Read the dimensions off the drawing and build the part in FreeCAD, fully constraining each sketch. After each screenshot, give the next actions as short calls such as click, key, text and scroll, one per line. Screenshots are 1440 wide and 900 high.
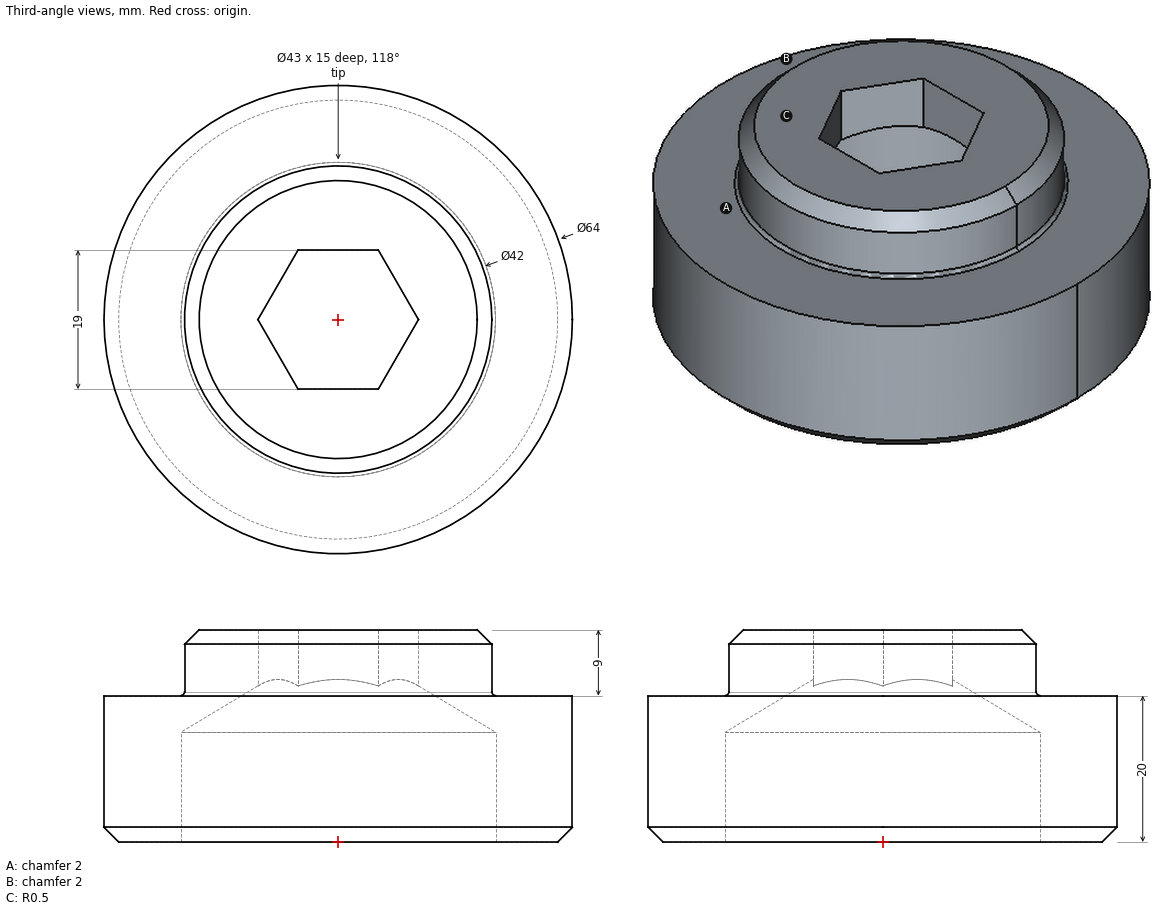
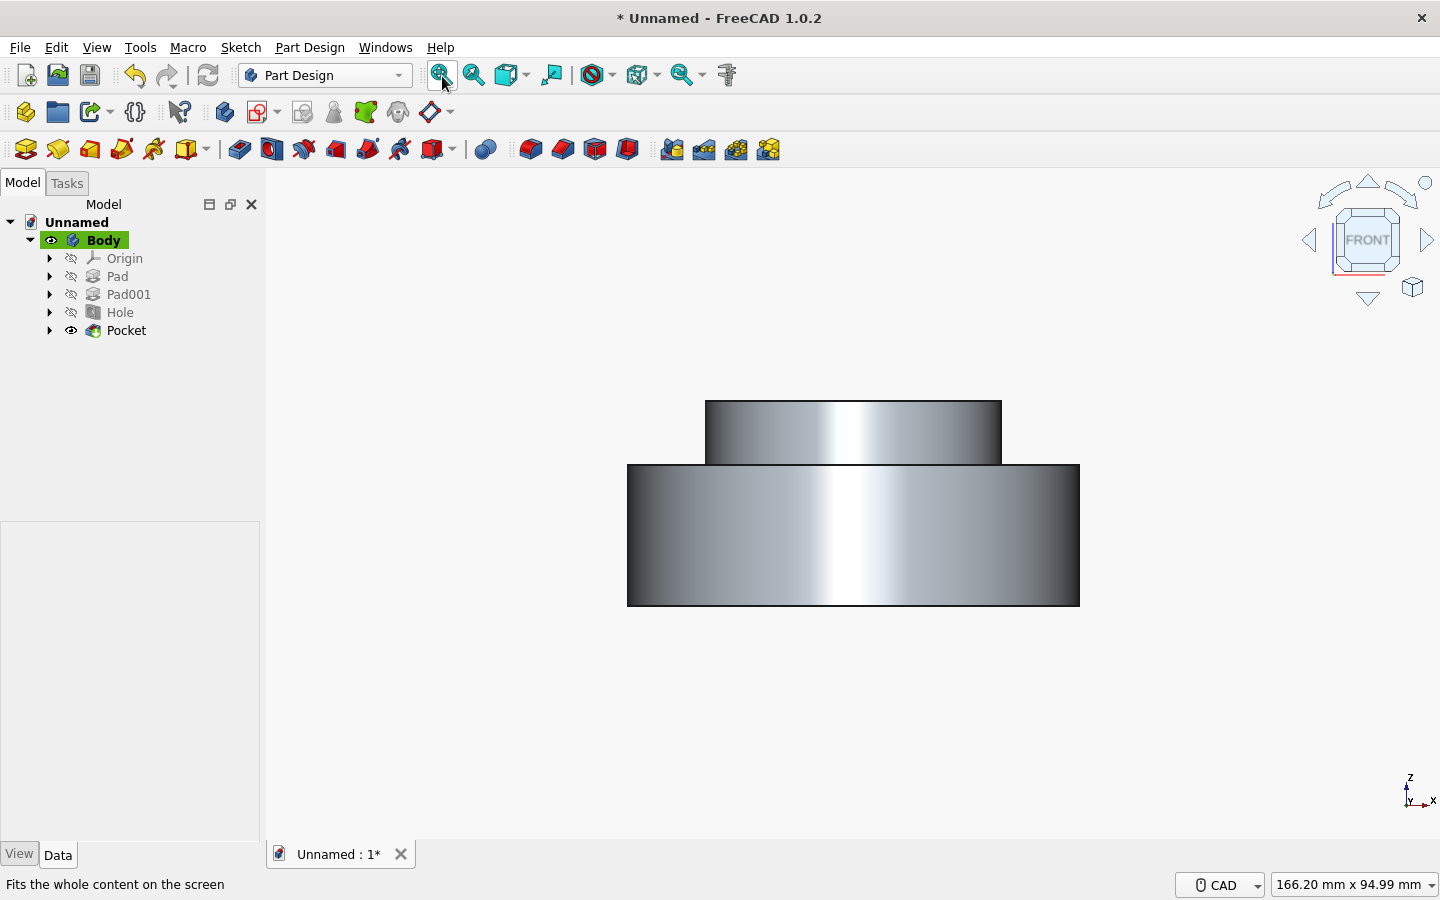
click(670, 605)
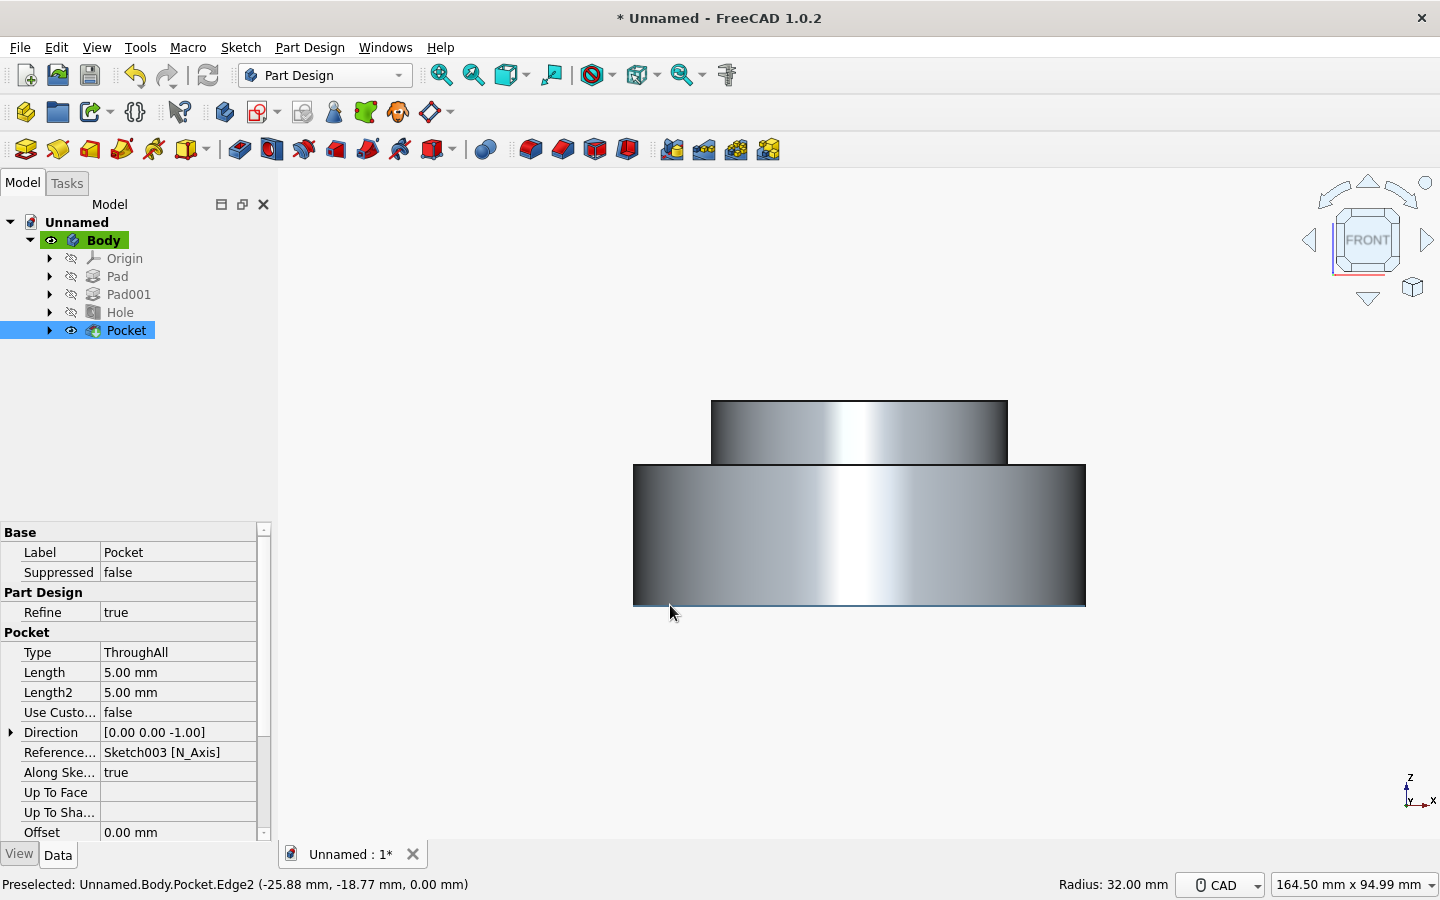
click(564, 150)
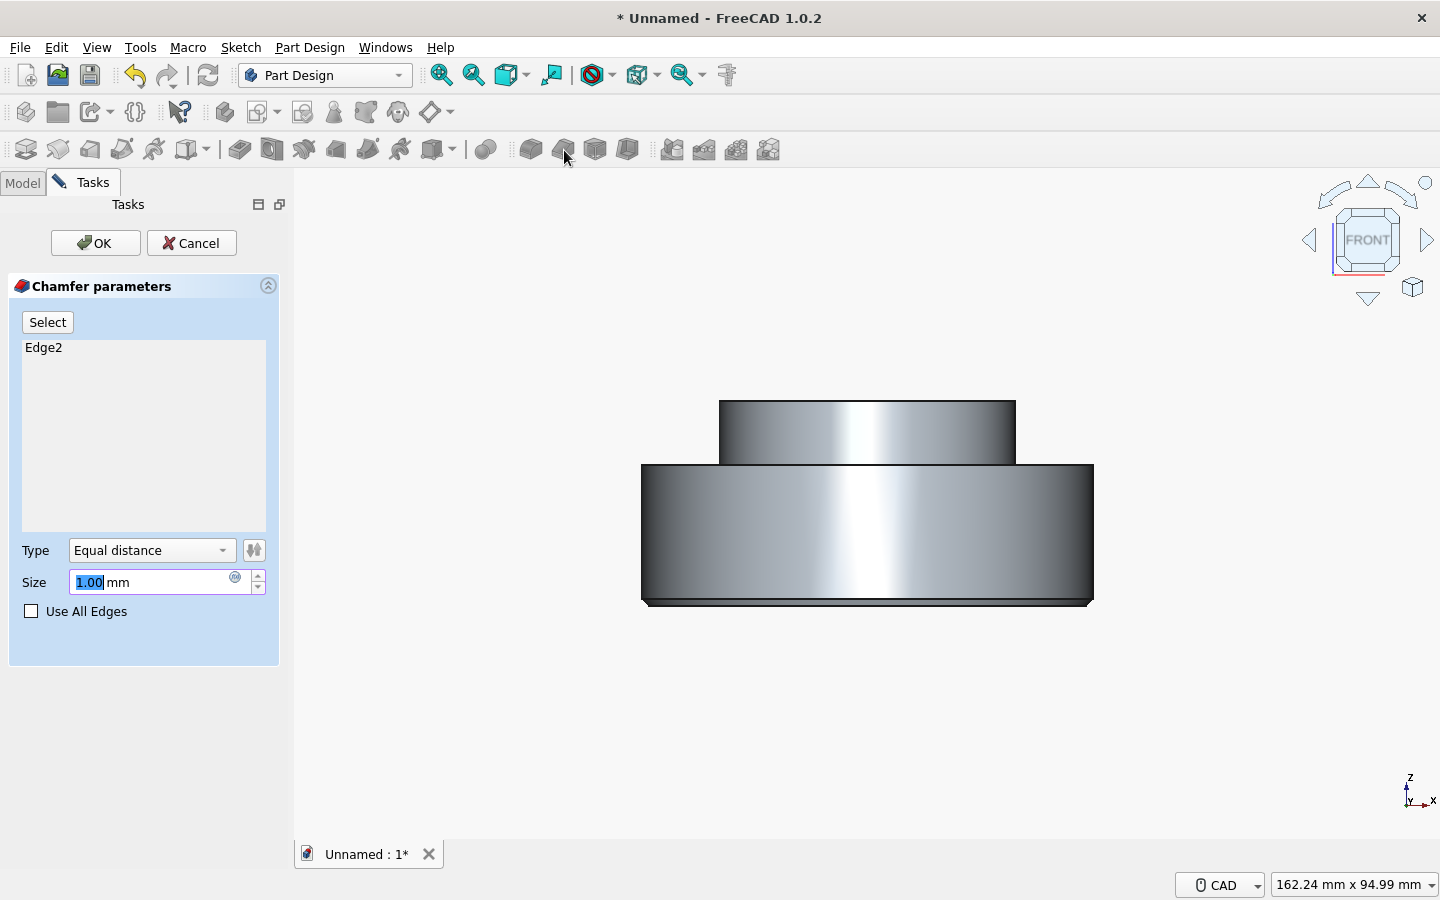
text(2)
key(Tab)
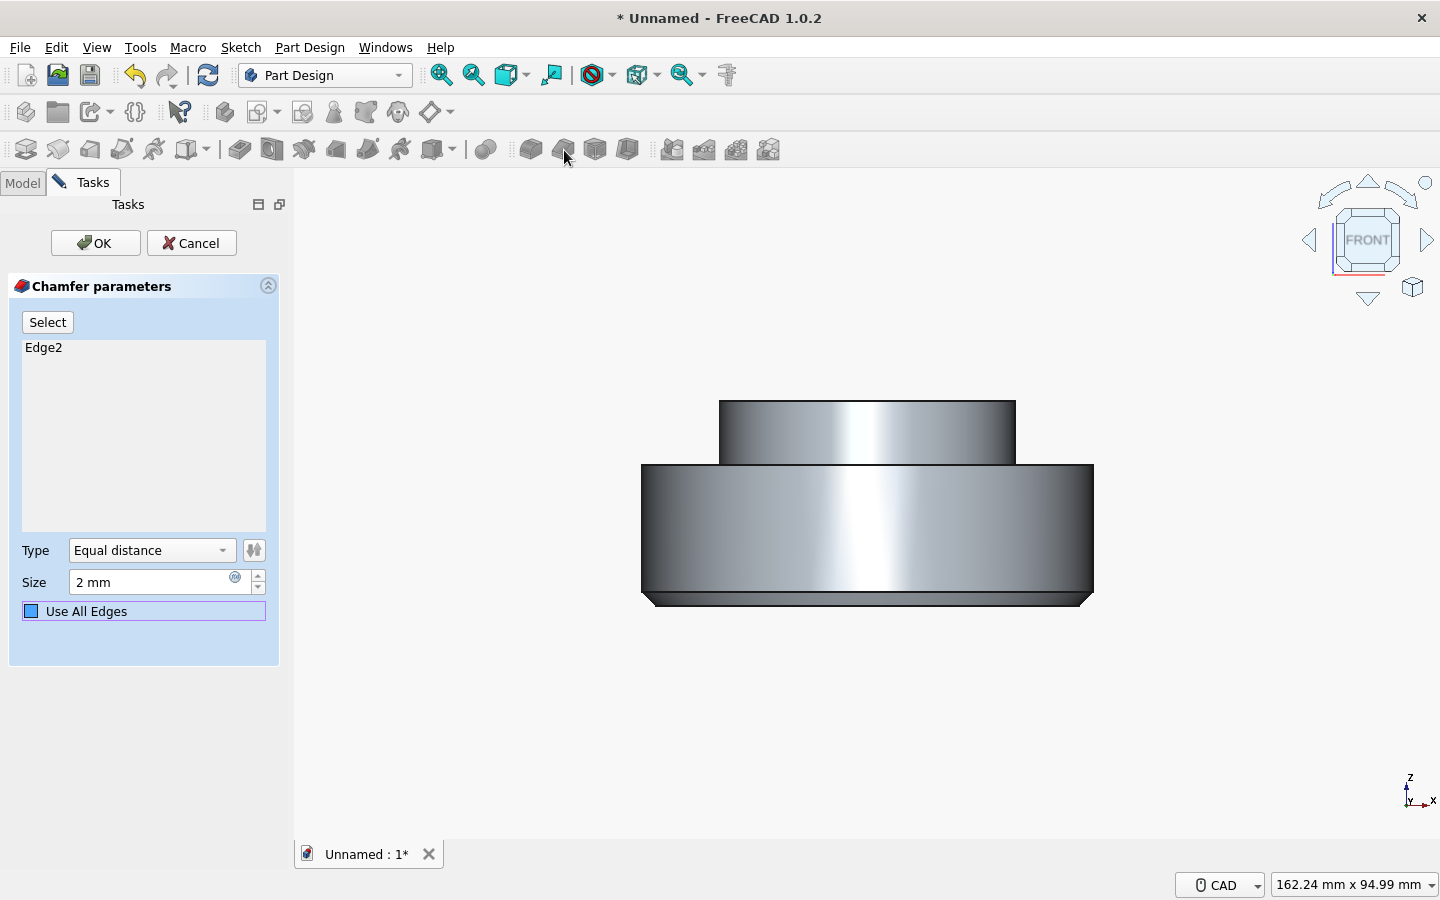
click(96, 243)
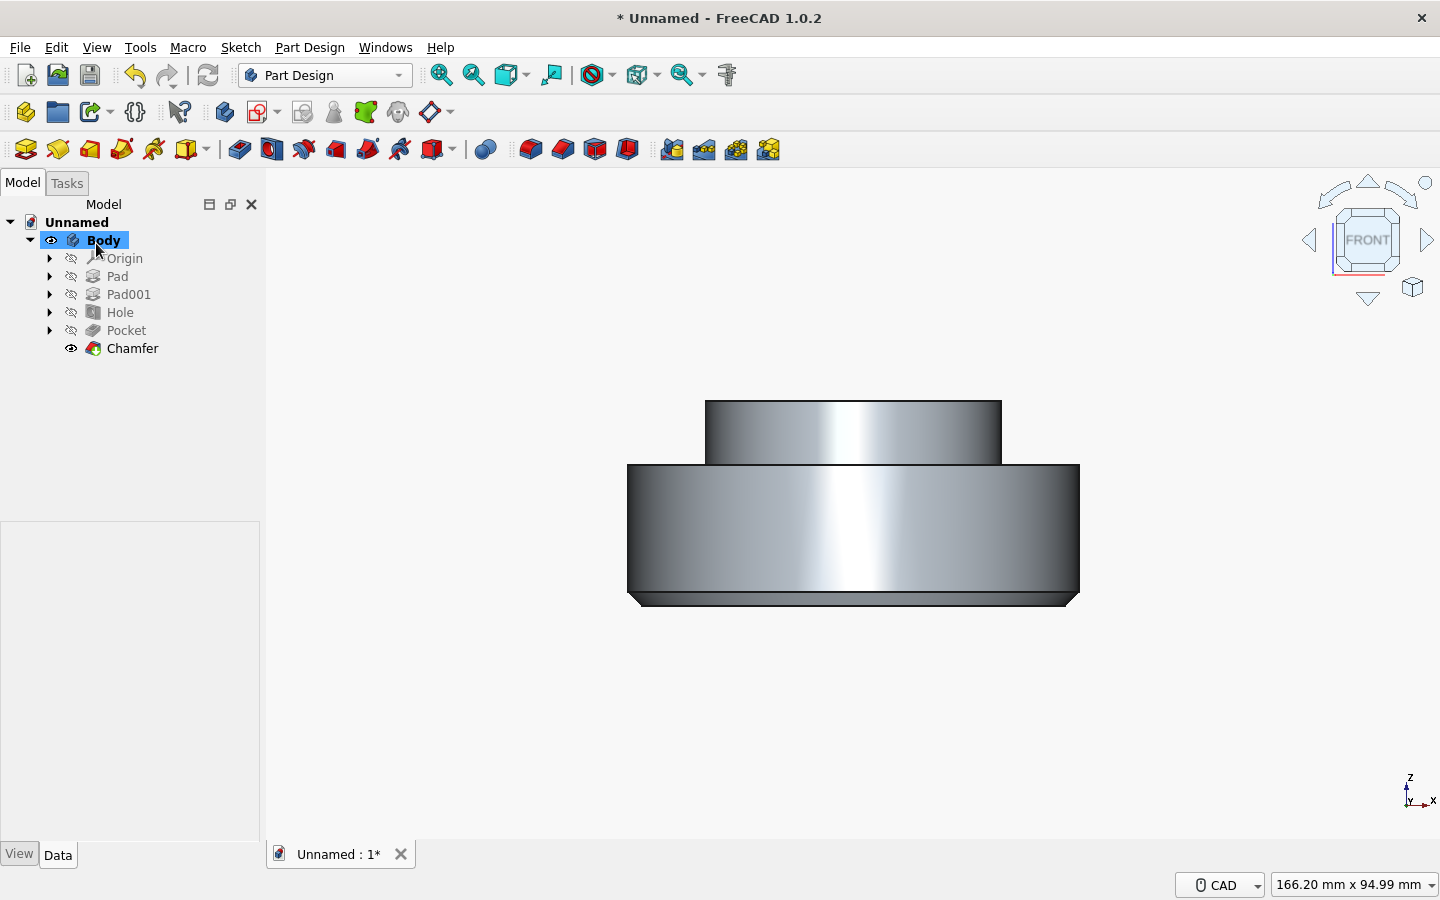
click(442, 76)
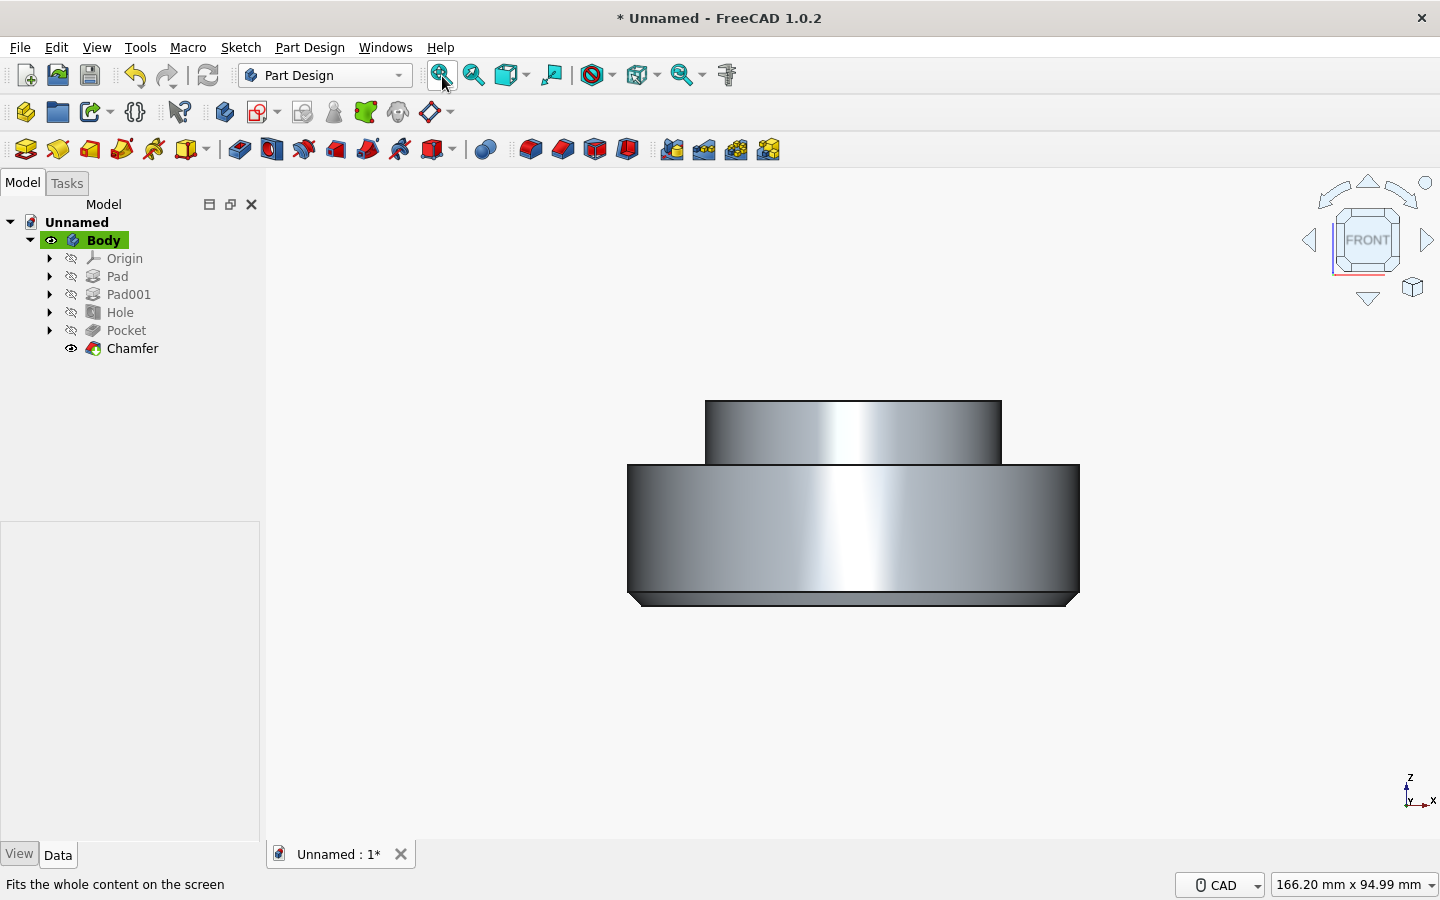
click(733, 400)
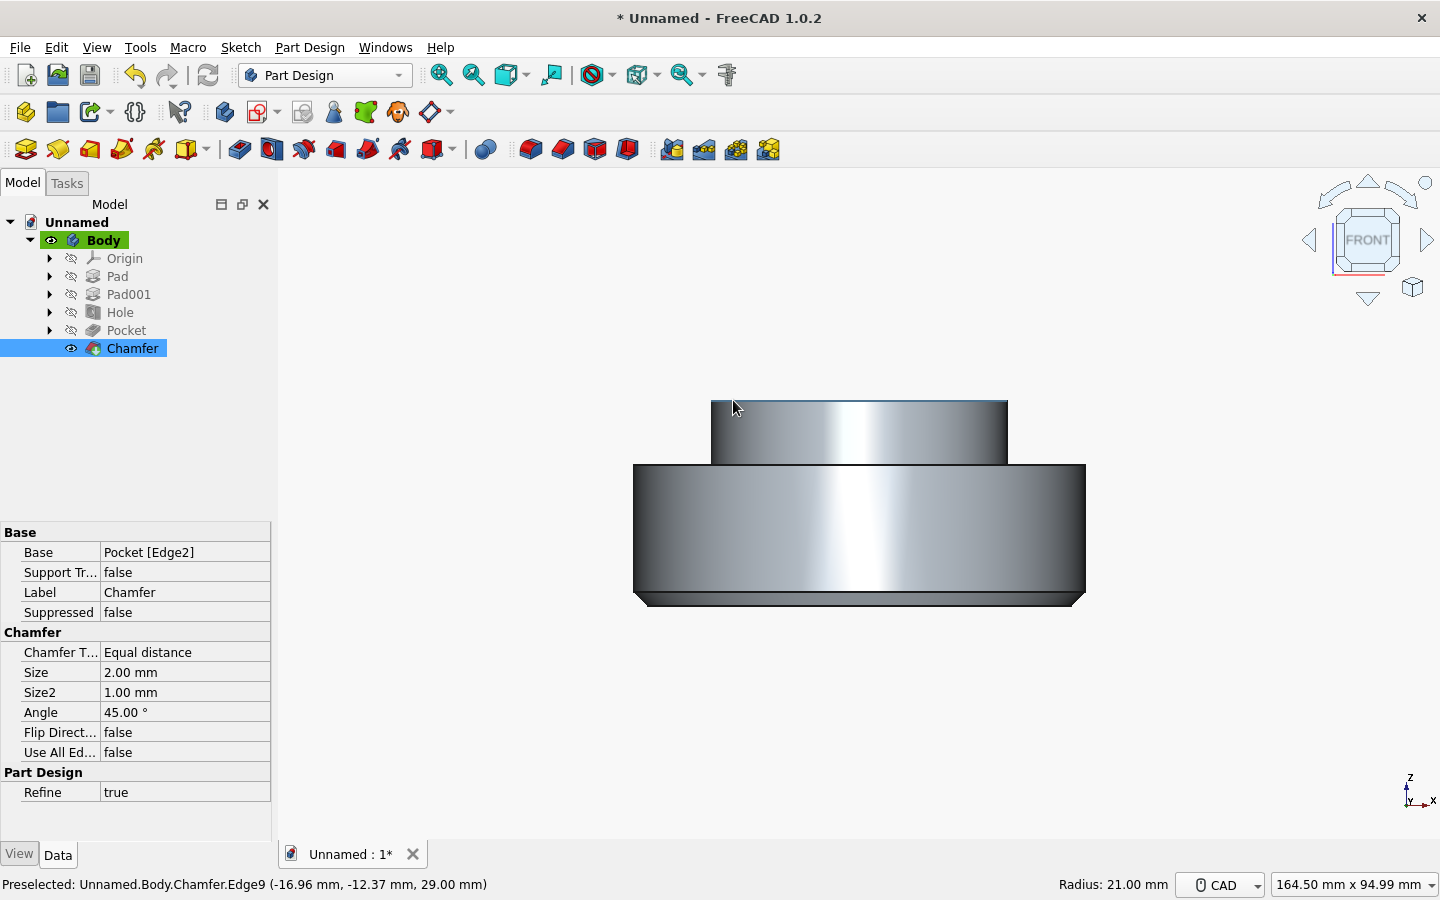
click(564, 150)